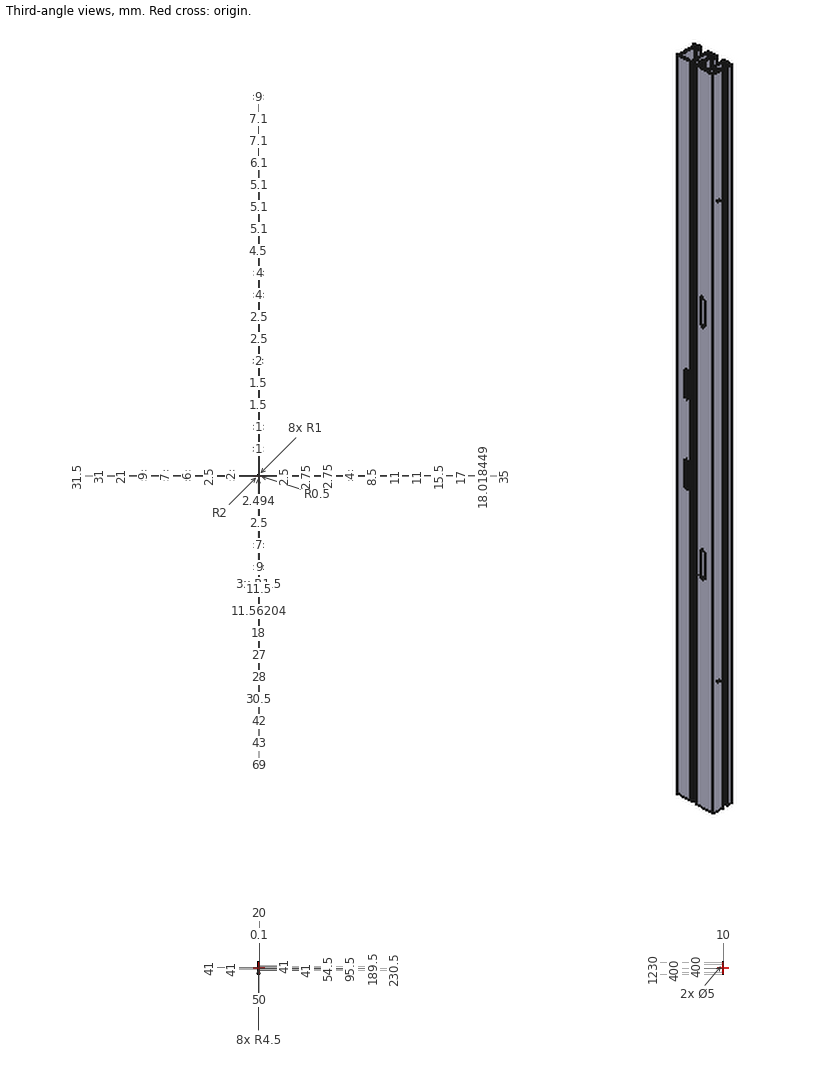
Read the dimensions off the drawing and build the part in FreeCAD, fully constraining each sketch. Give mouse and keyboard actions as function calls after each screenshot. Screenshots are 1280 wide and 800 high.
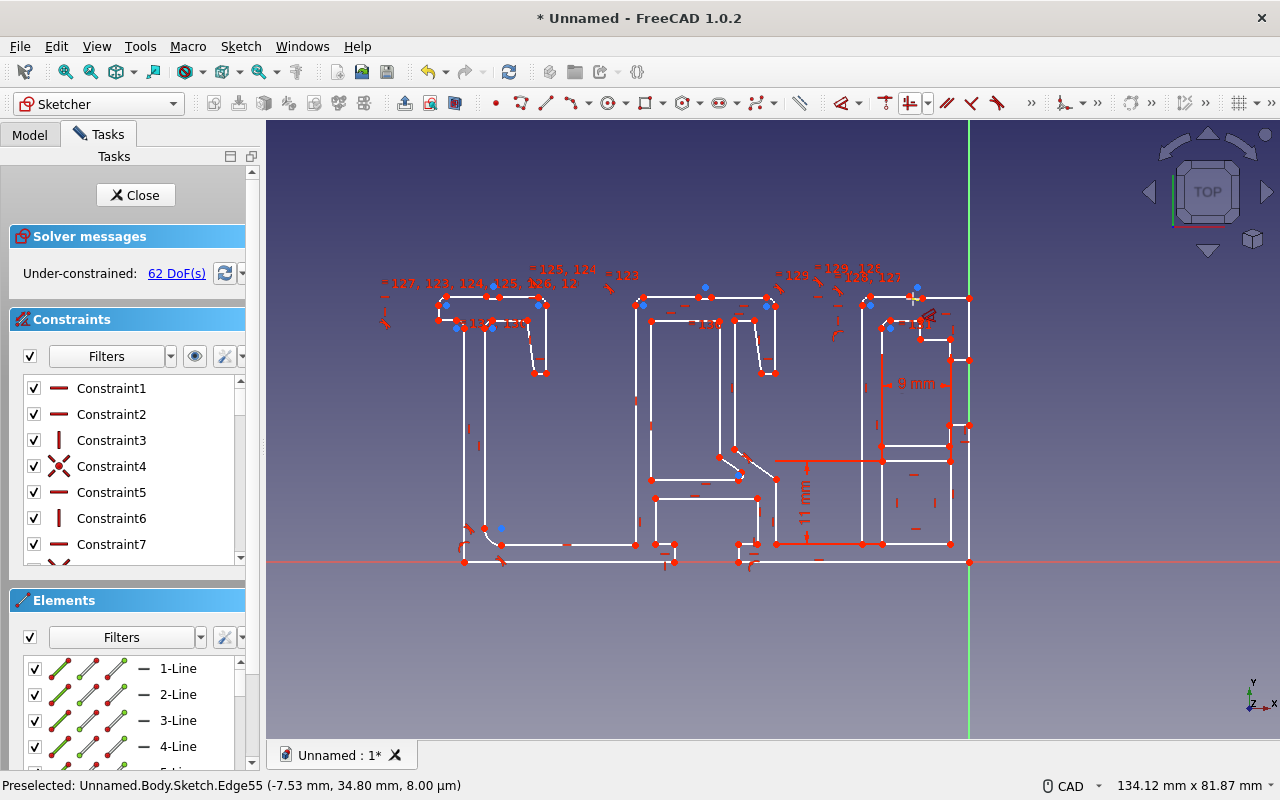
scroll(702, 299, up, 7)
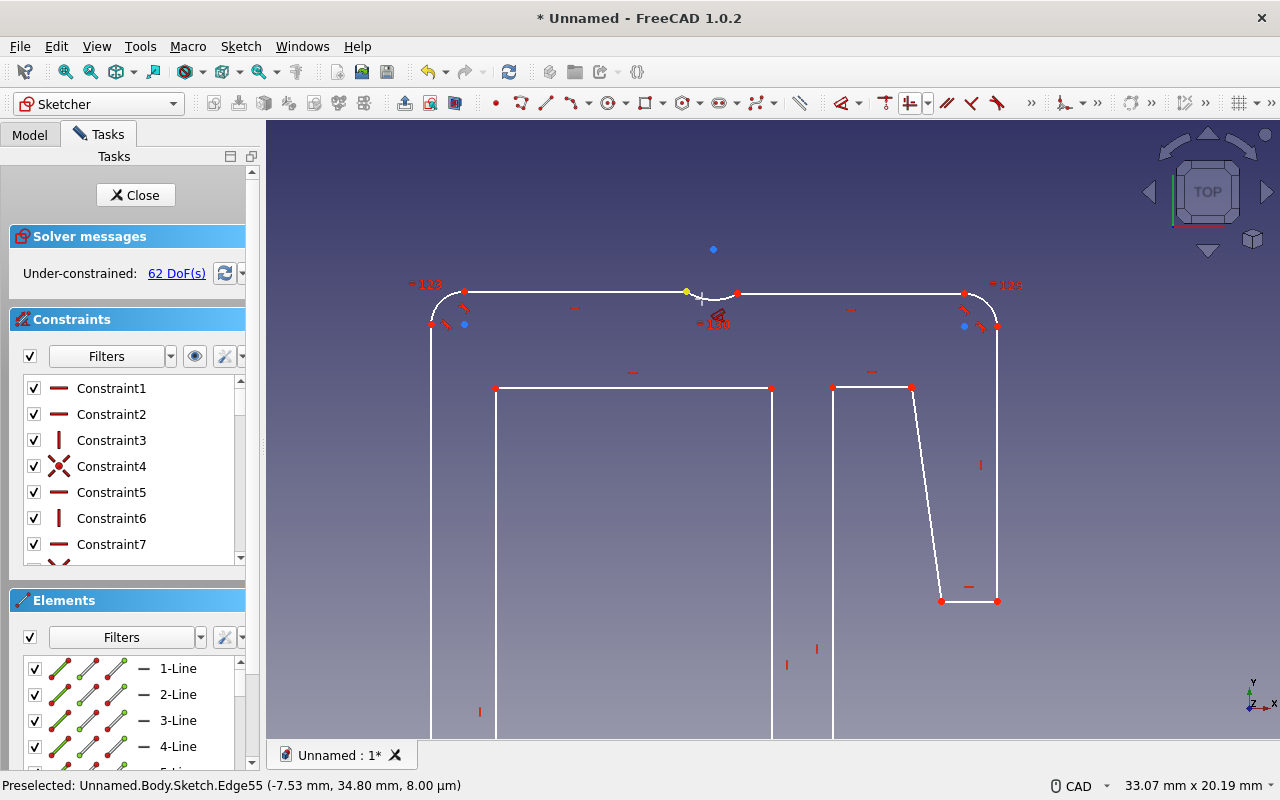
click(702, 298)
click(694, 329)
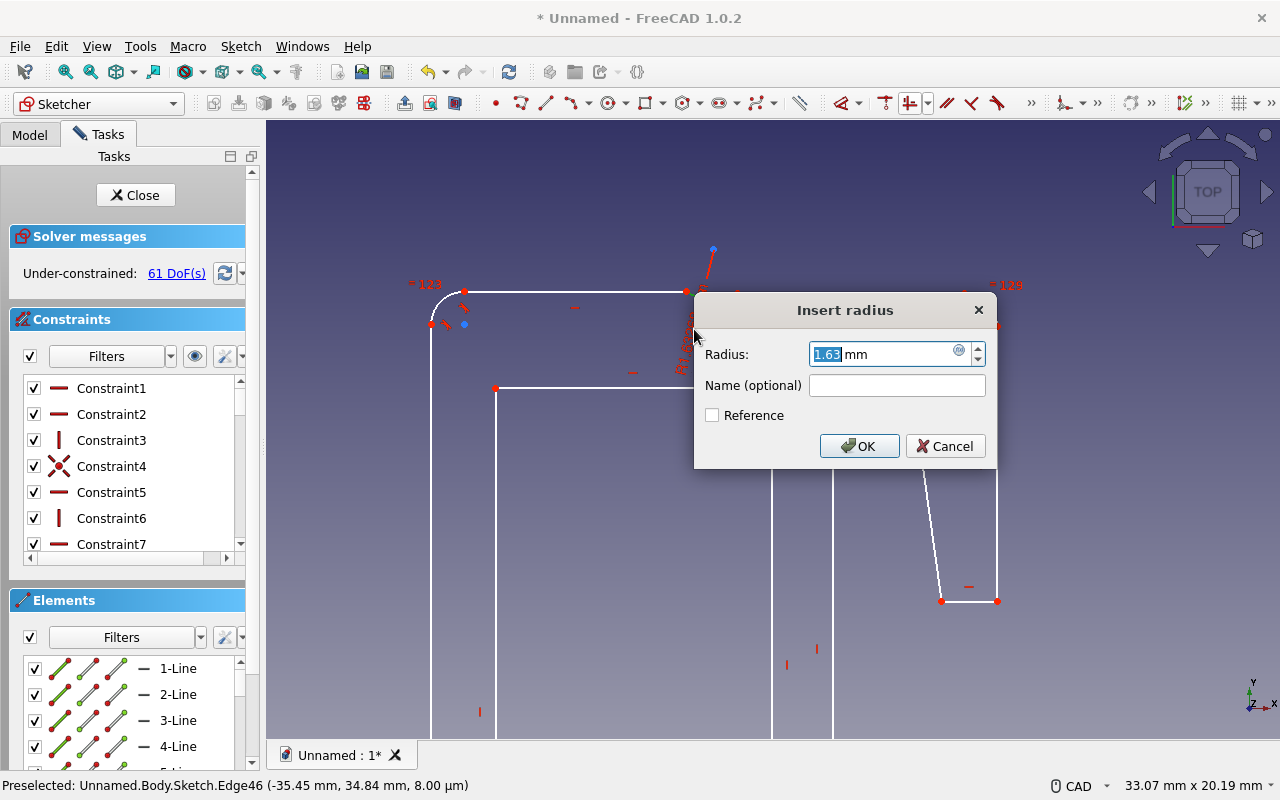
text(1.5)
key(Return)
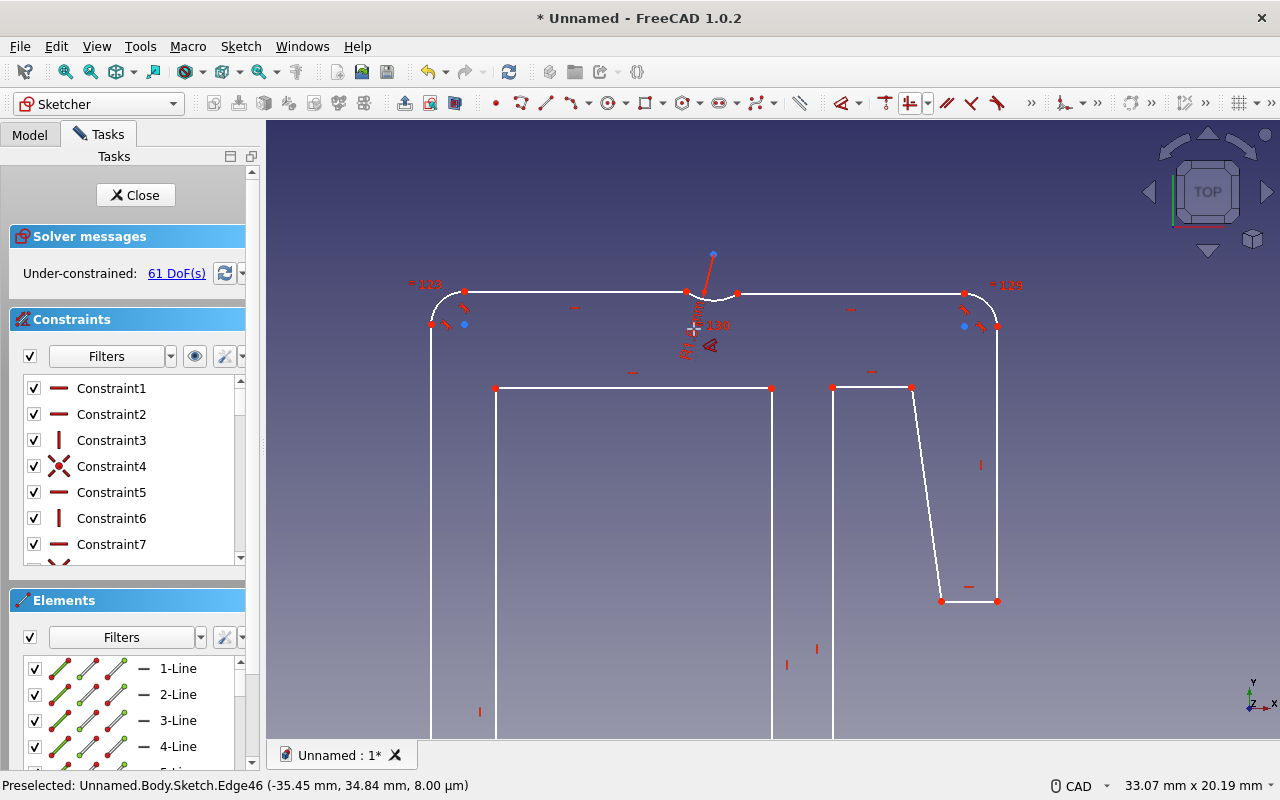
scroll(449, 296, up, 2)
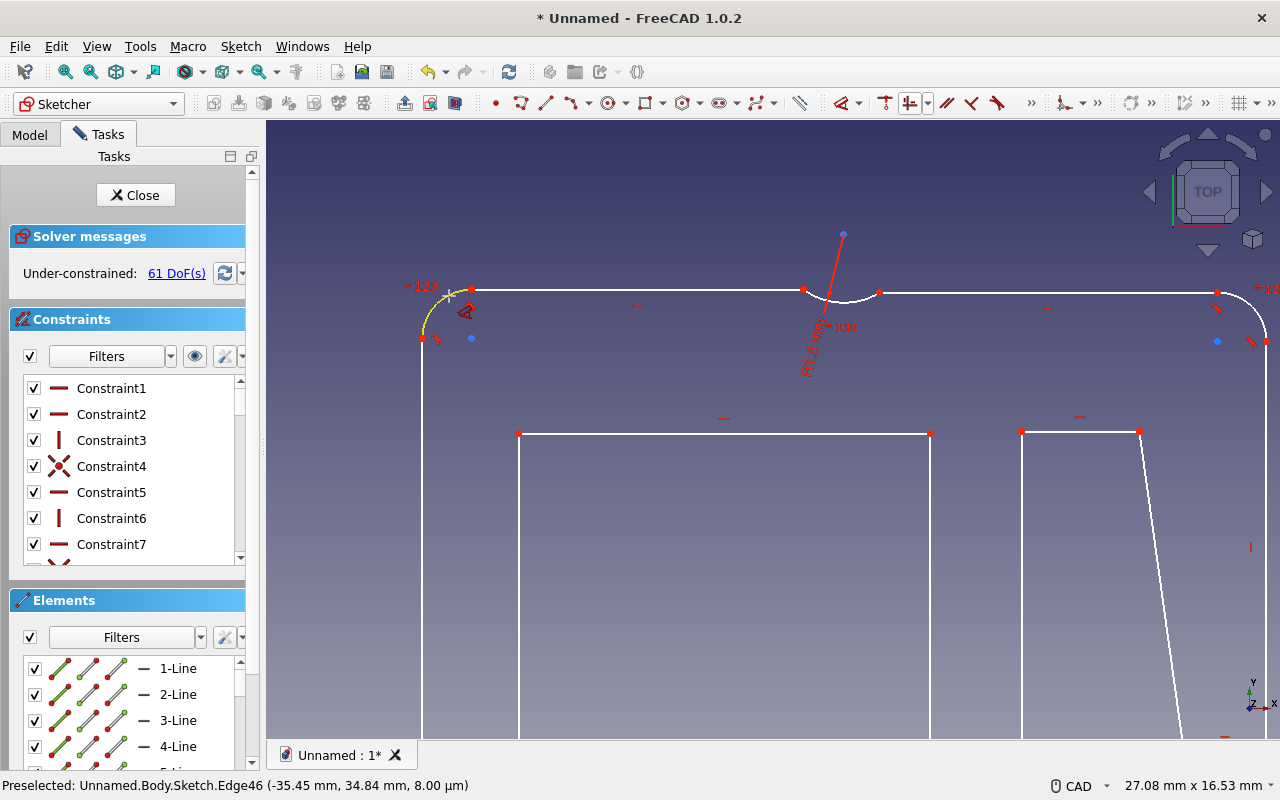
click(449, 295)
click(434, 266)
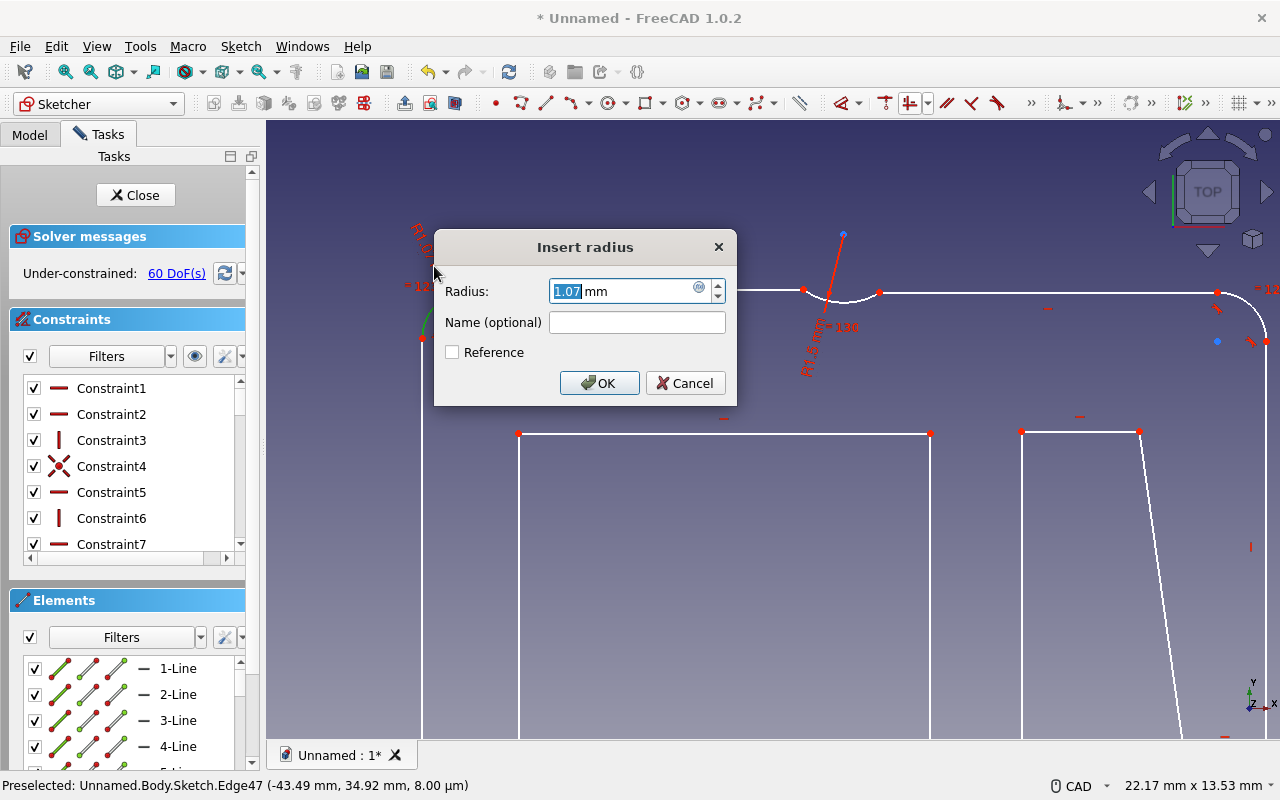
text(1)
key(Return)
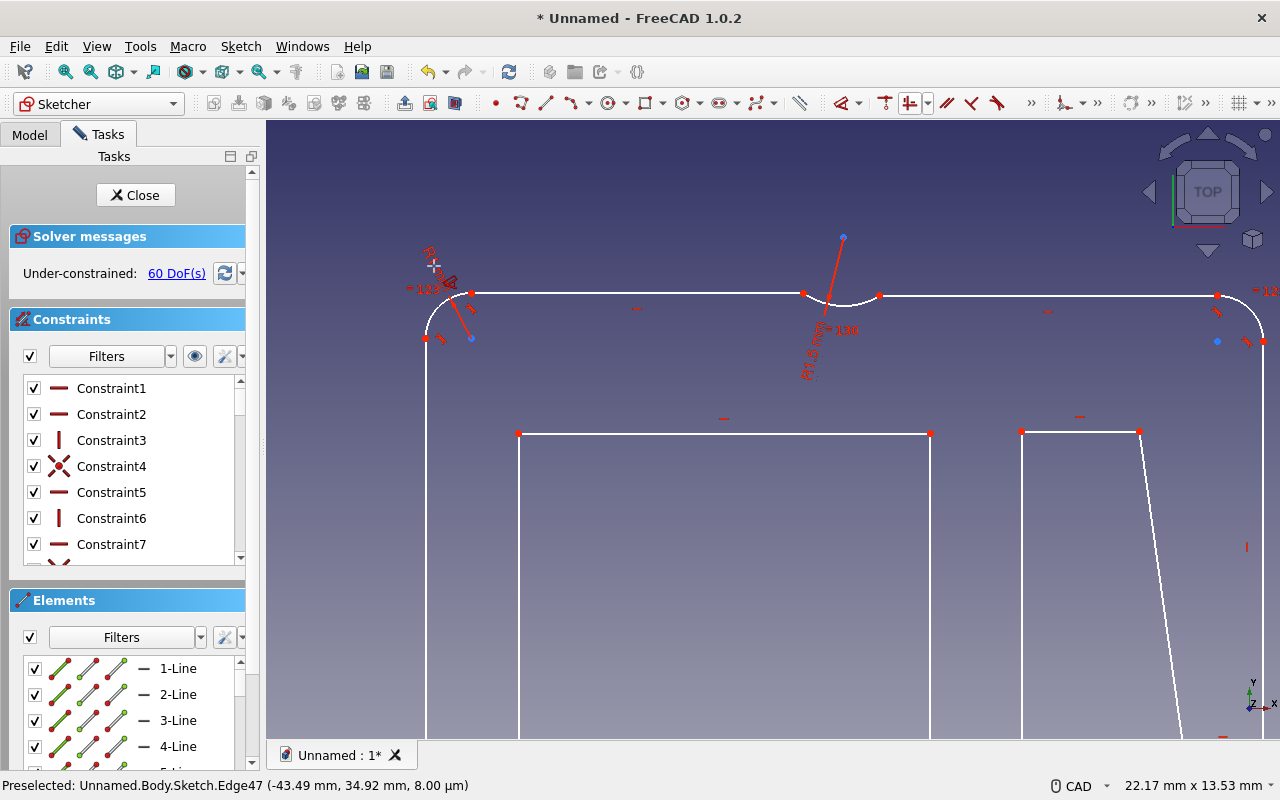
scroll(678, 299, down, 9)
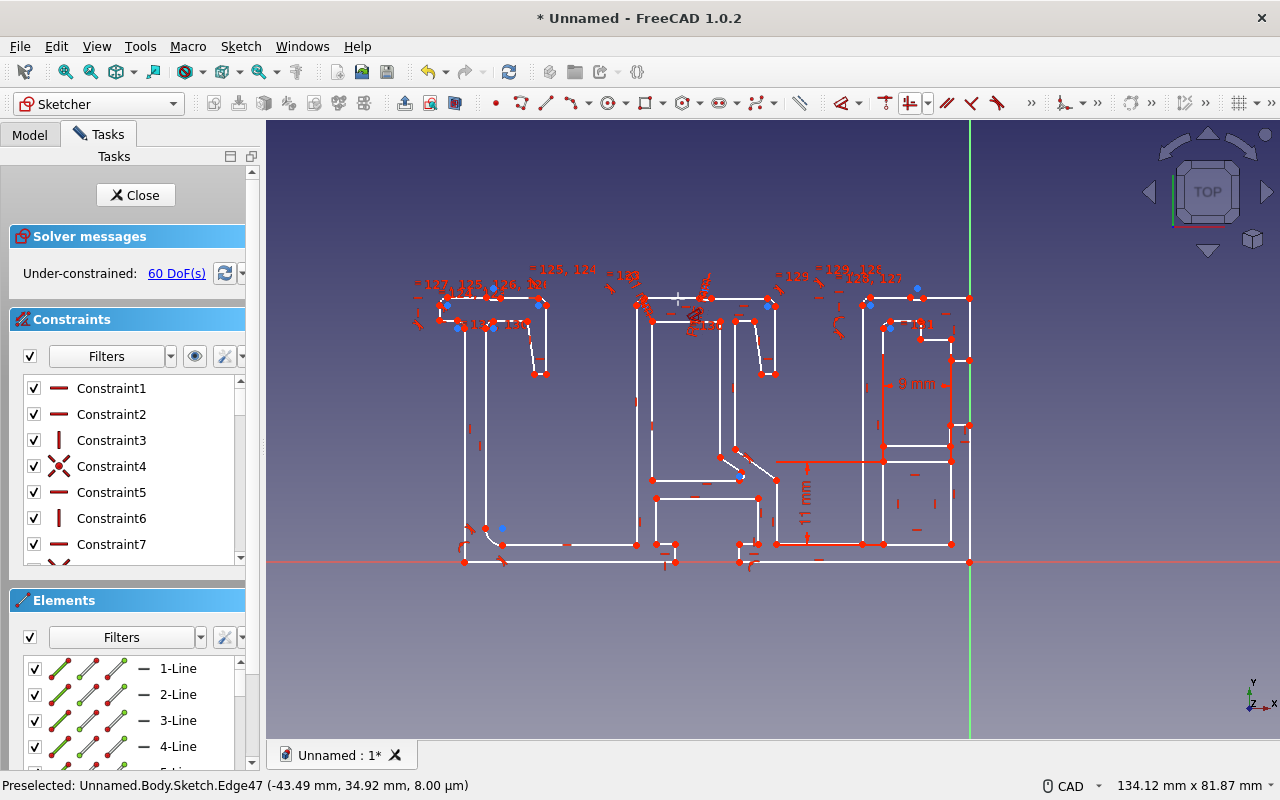
scroll(488, 536, up, 5)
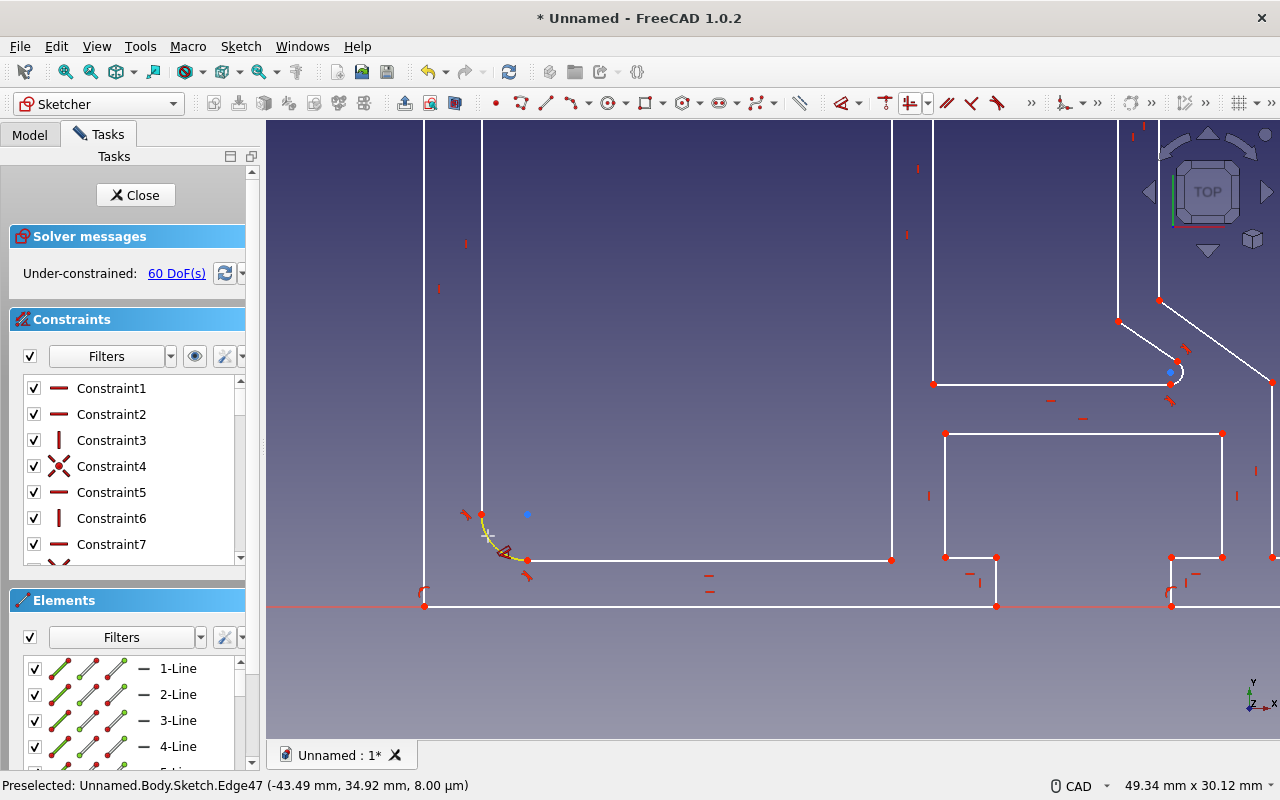
click(487, 535)
click(458, 549)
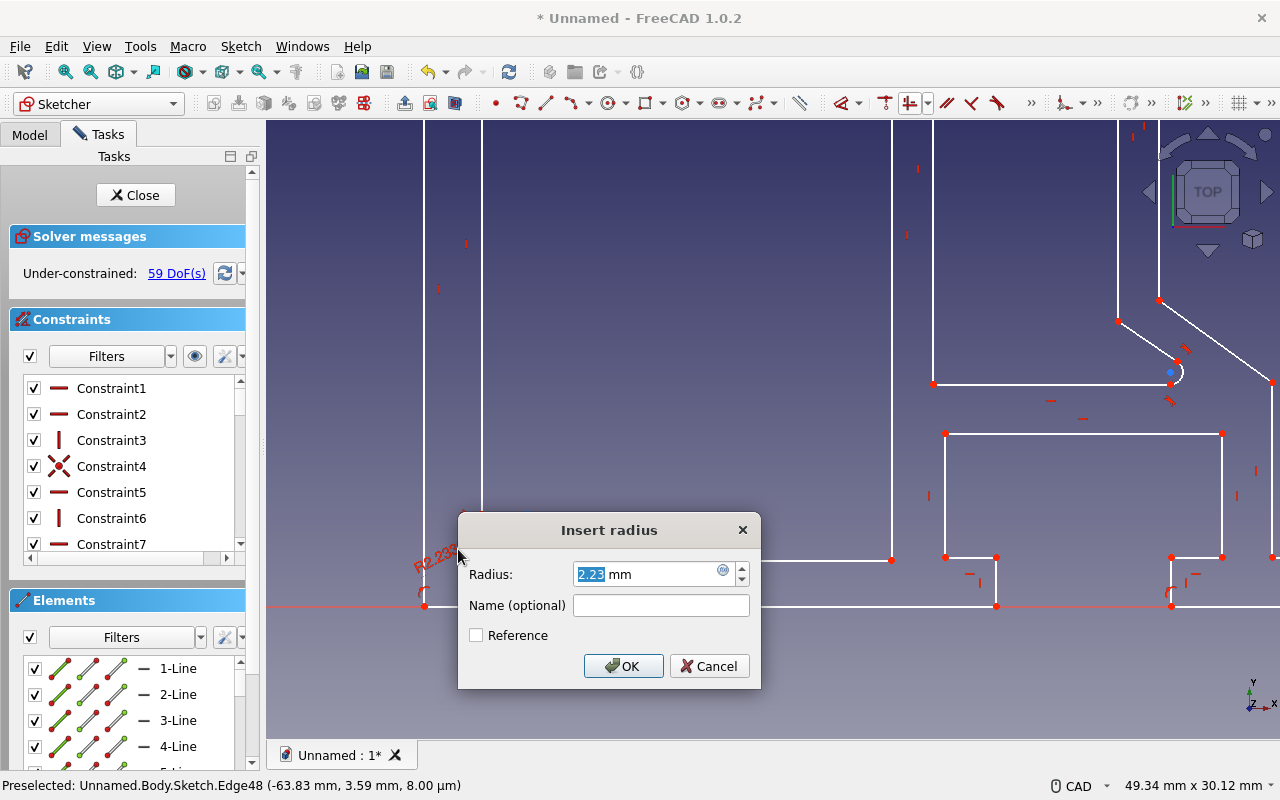
text(2)
key(Return)